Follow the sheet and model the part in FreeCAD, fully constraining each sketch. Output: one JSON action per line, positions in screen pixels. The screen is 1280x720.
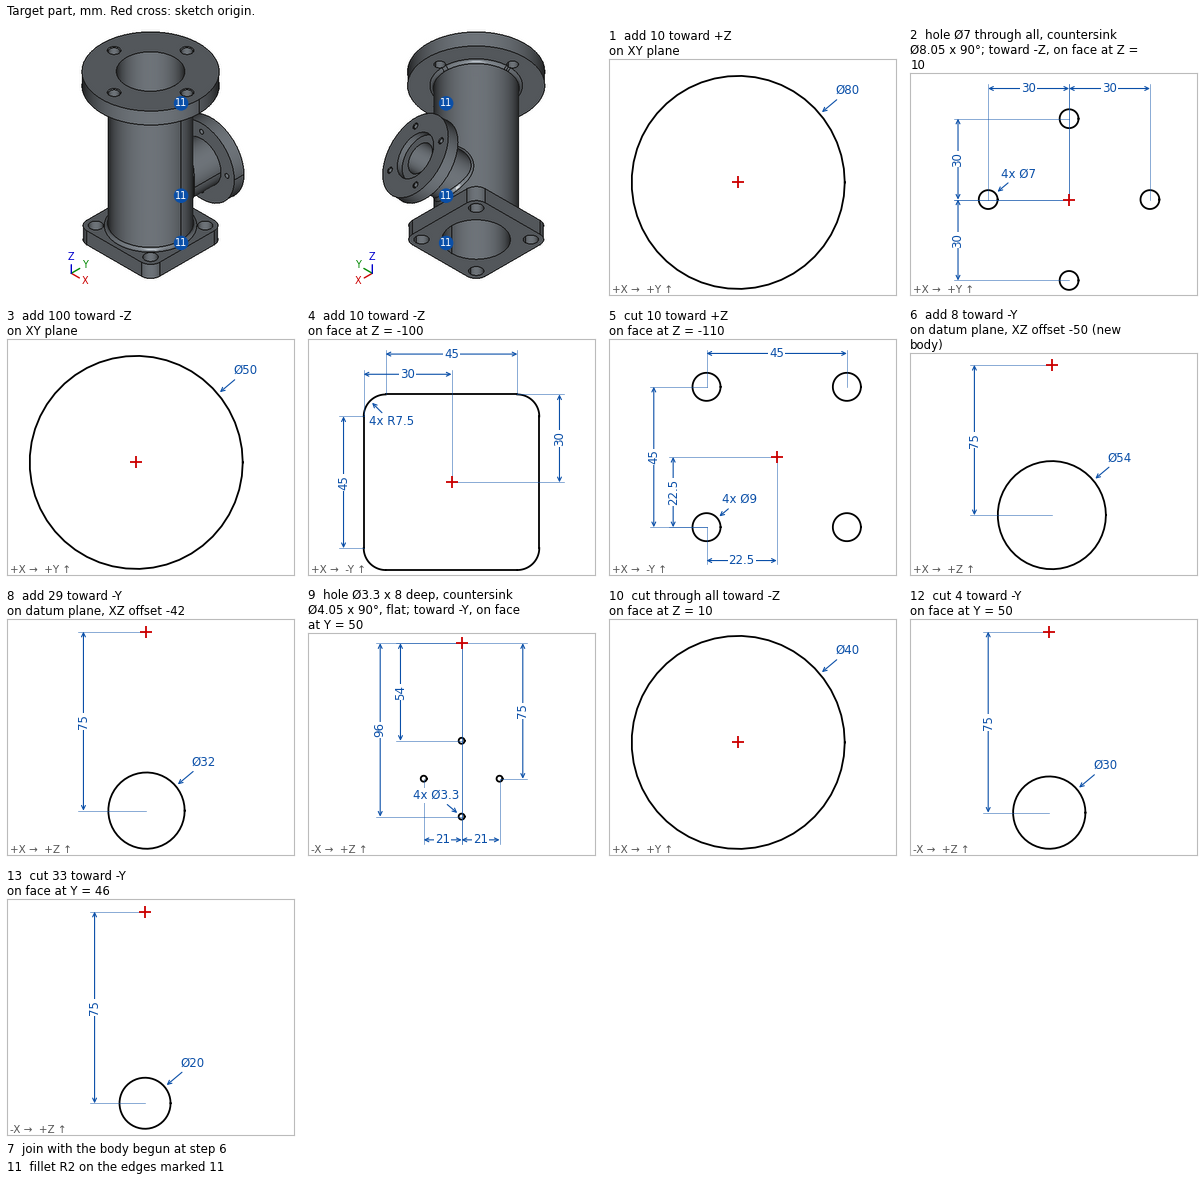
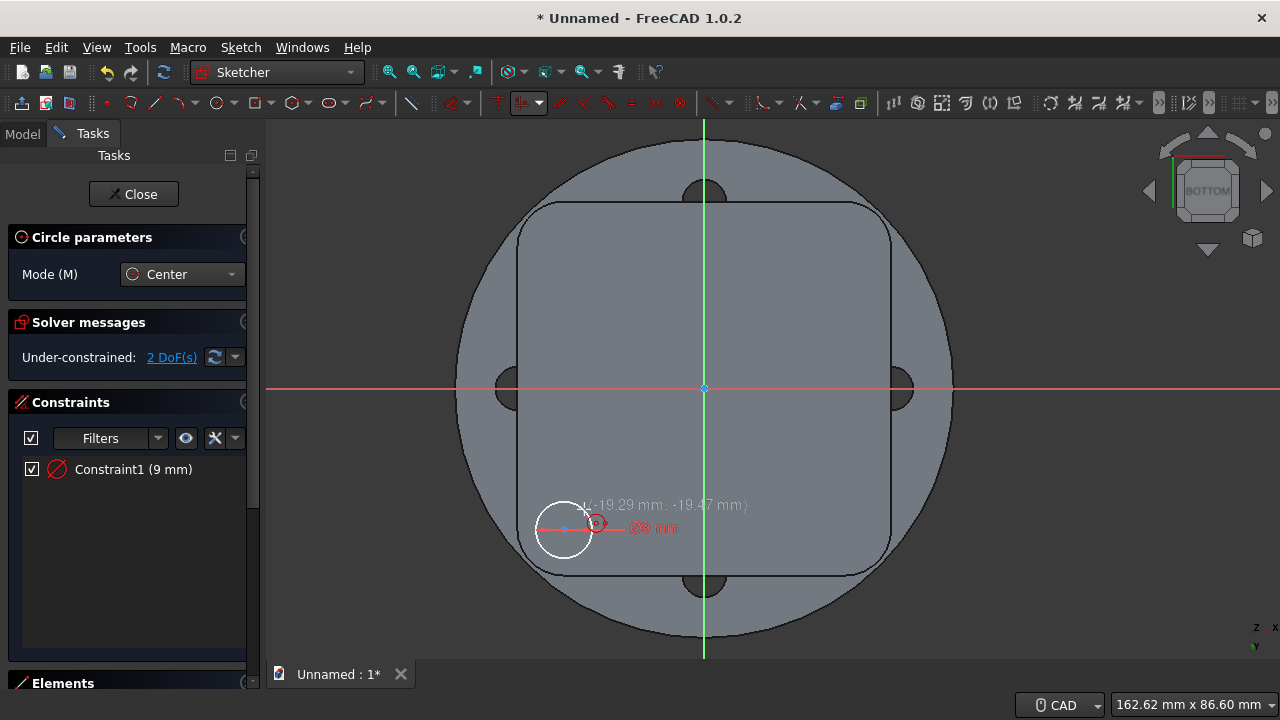
{"action": "left_click", "coordinate": [564, 248]}
{"action": "mouse_move", "coordinate": [584, 228]}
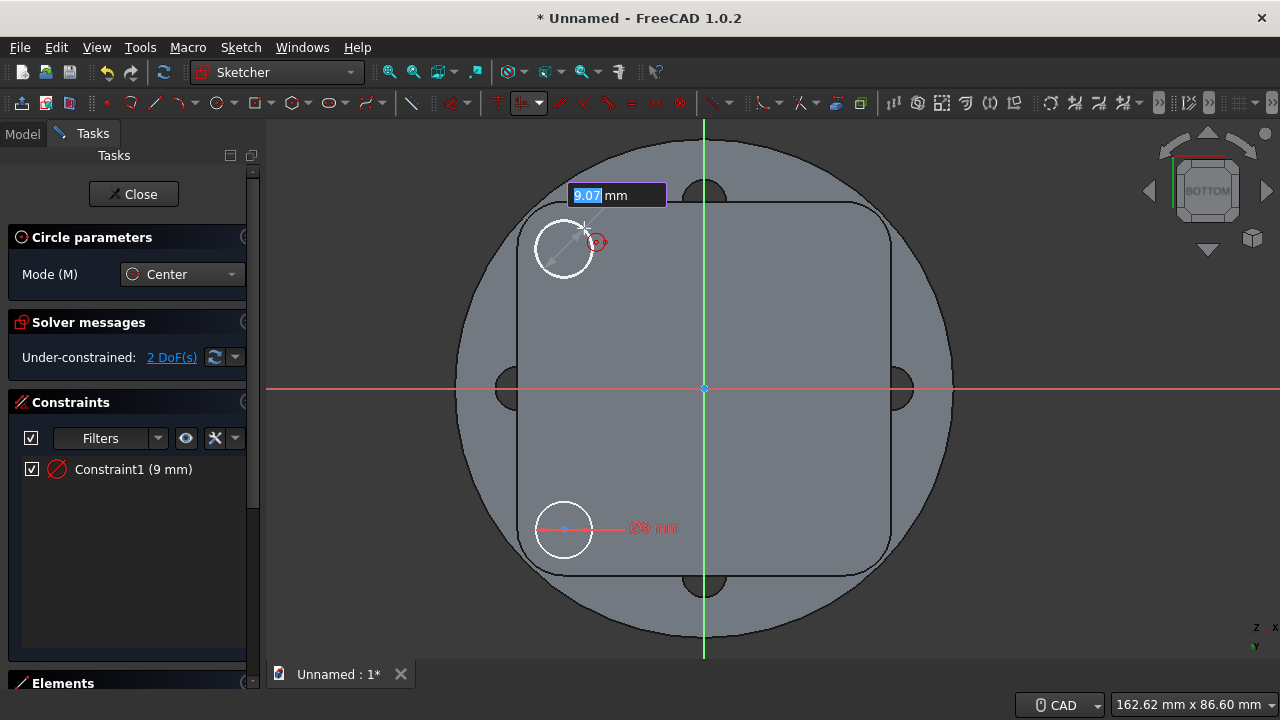
{"action": "type", "text": "9"}
{"action": "key", "text": "Return"}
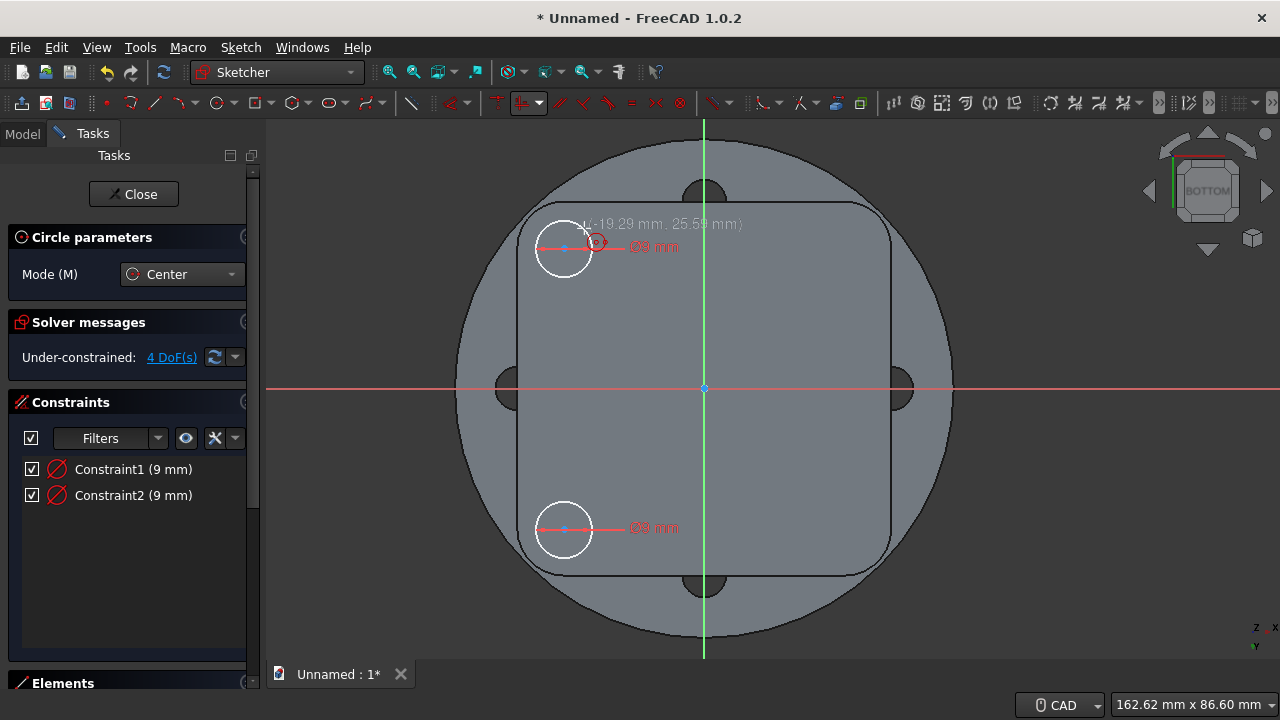
{"action": "left_click", "coordinate": [845, 248]}
{"action": "mouse_move", "coordinate": [864, 228]}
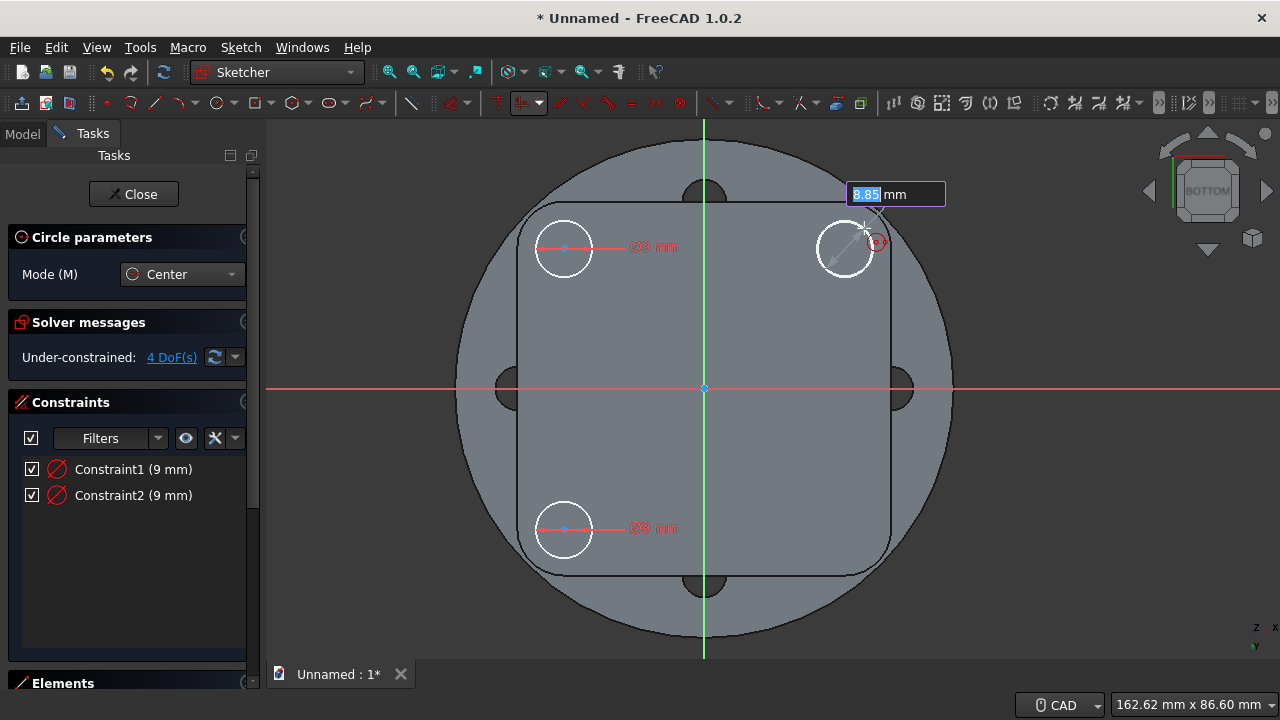
{"action": "type", "text": "9"}
{"action": "key", "text": "Return"}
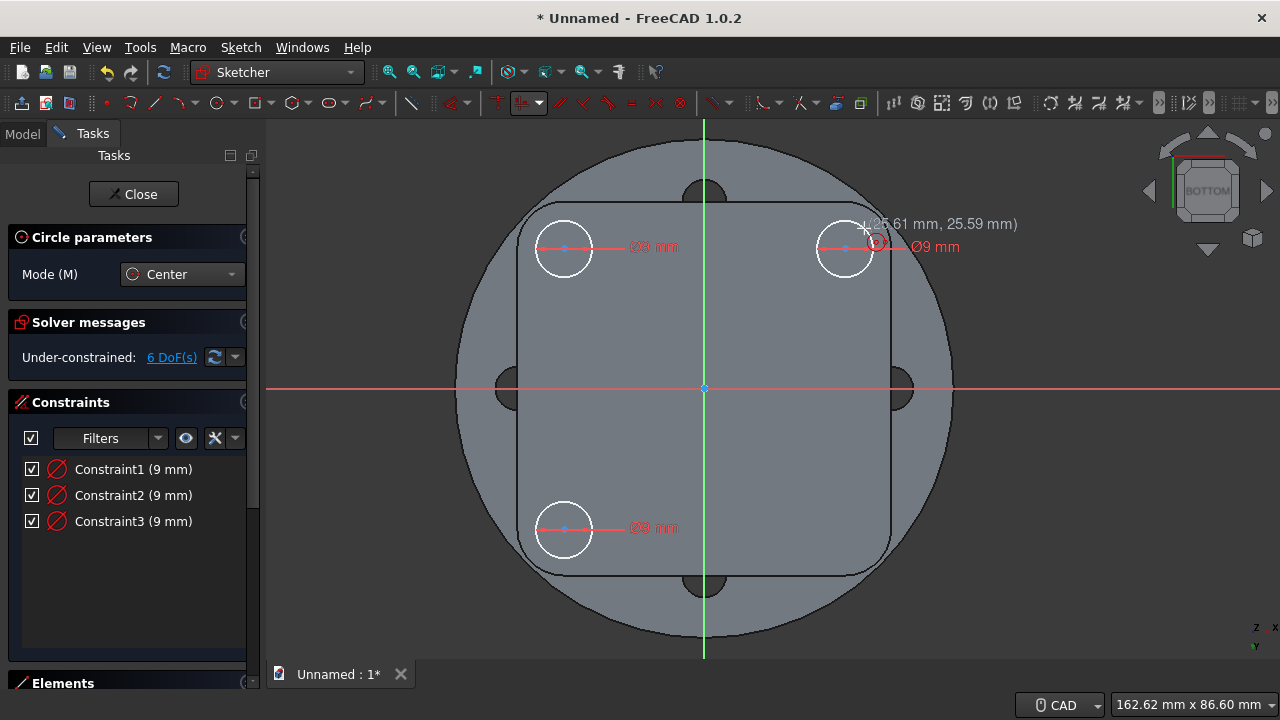
{"action": "left_click", "coordinate": [845, 529]}
{"action": "mouse_move", "coordinate": [864, 509]}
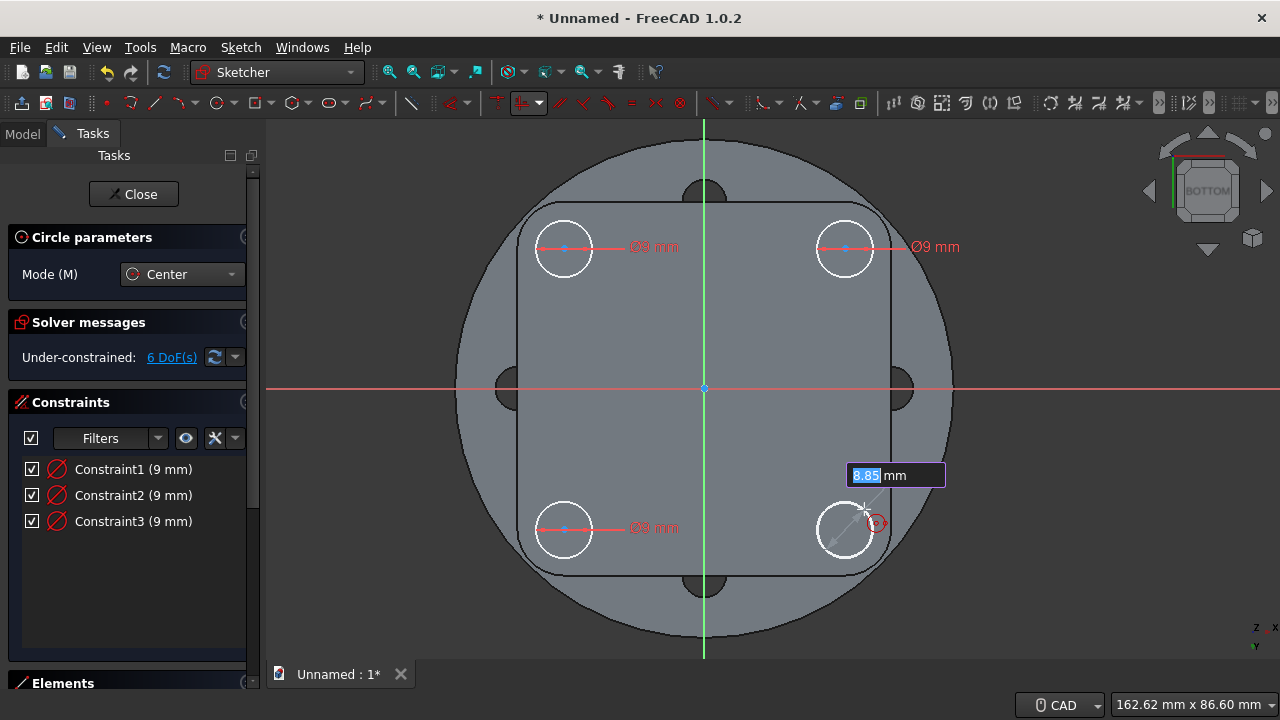
{"action": "type", "text": "9"}
{"action": "key", "text": "Return"}
{"action": "key", "text": "Escape"}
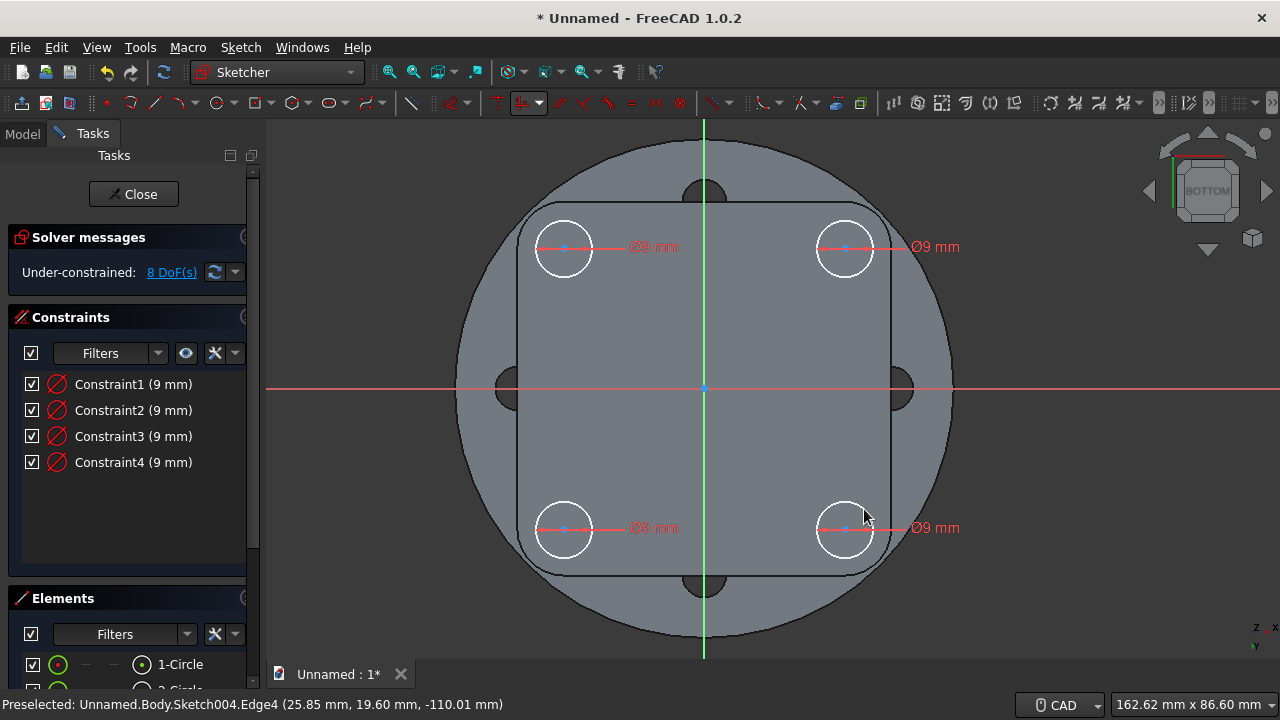
{"action": "left_click", "coordinate": [564, 530]}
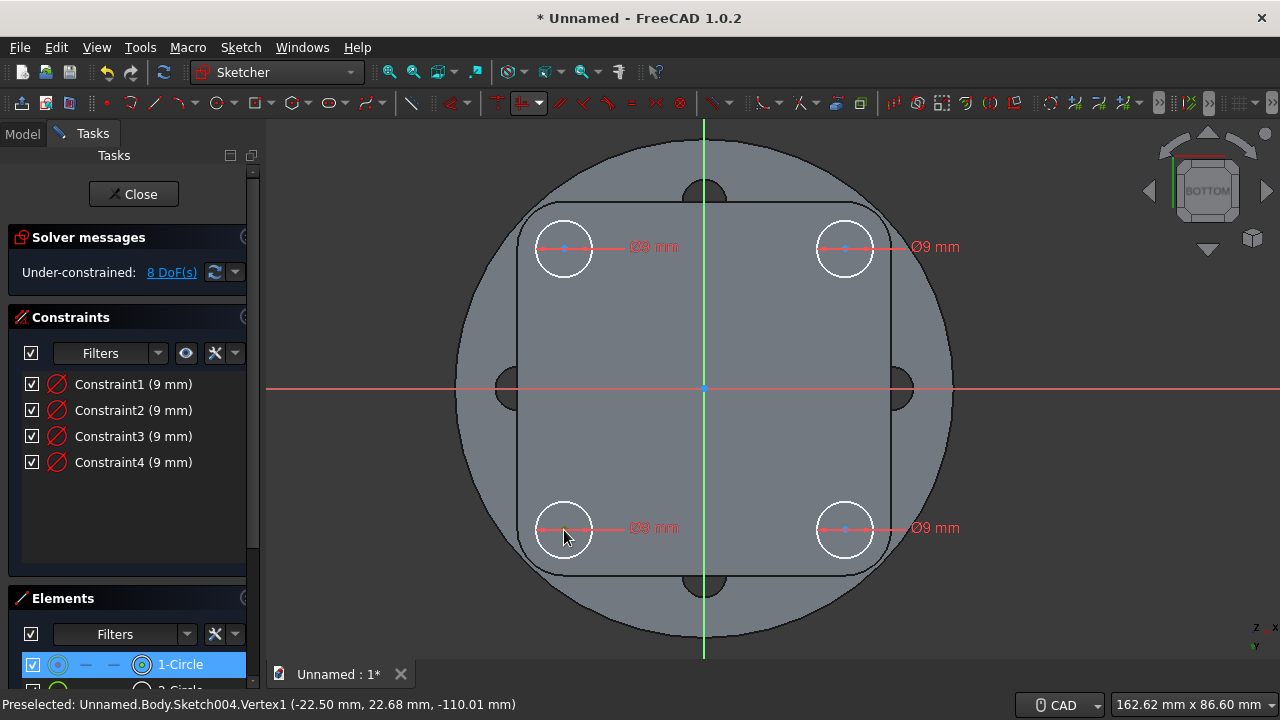
{"action": "left_click", "coordinate": [564, 249]}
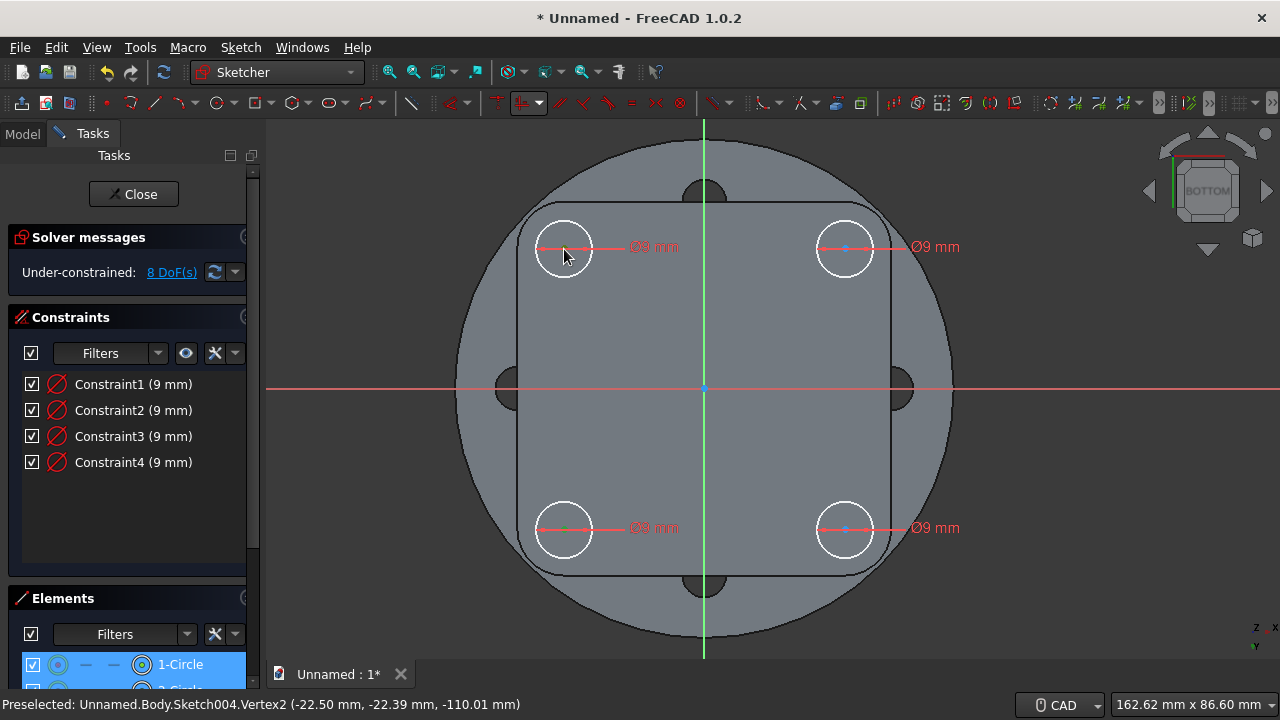
{"action": "left_click", "coordinate": [542, 104]}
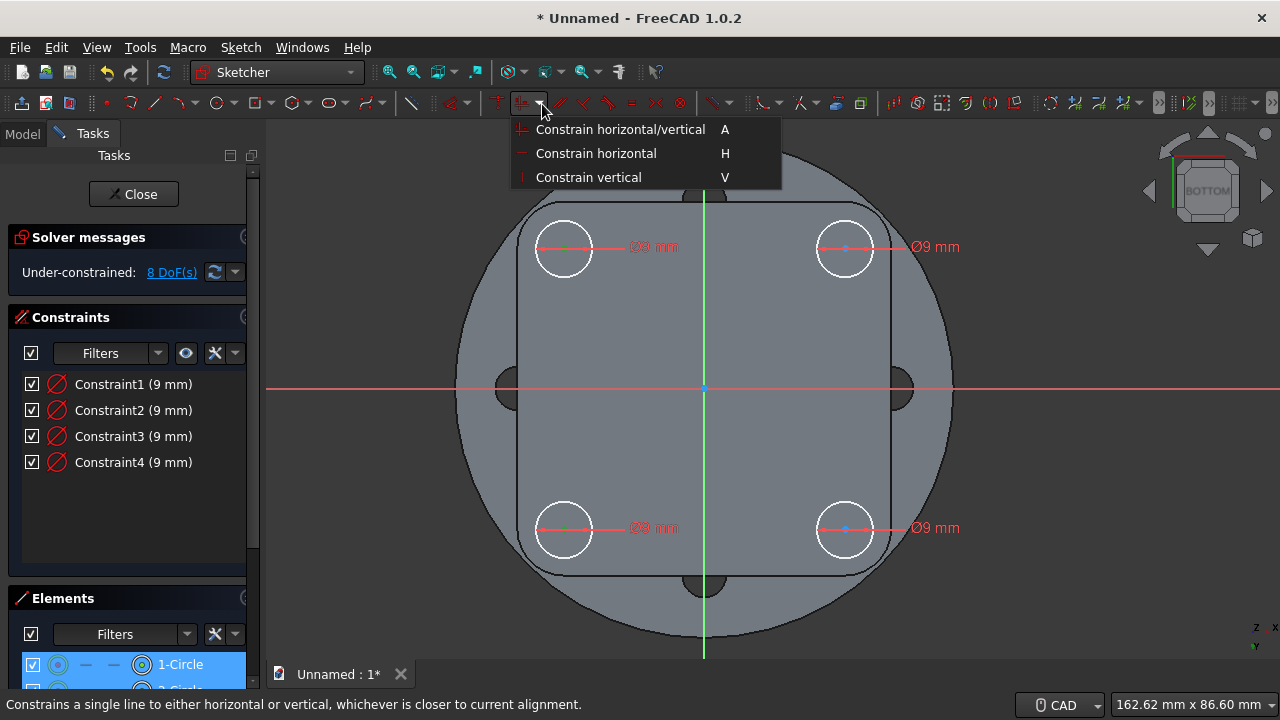
{"action": "left_click", "coordinate": [646, 177]}